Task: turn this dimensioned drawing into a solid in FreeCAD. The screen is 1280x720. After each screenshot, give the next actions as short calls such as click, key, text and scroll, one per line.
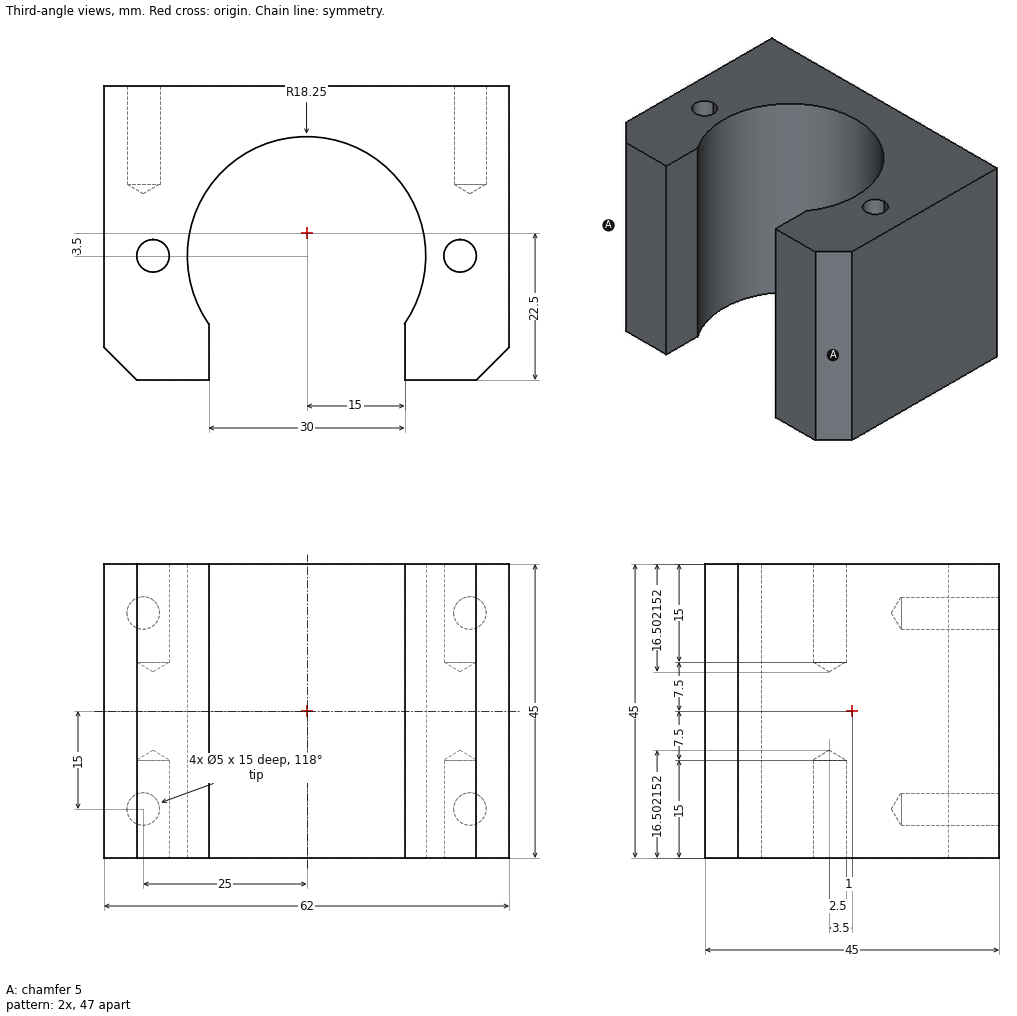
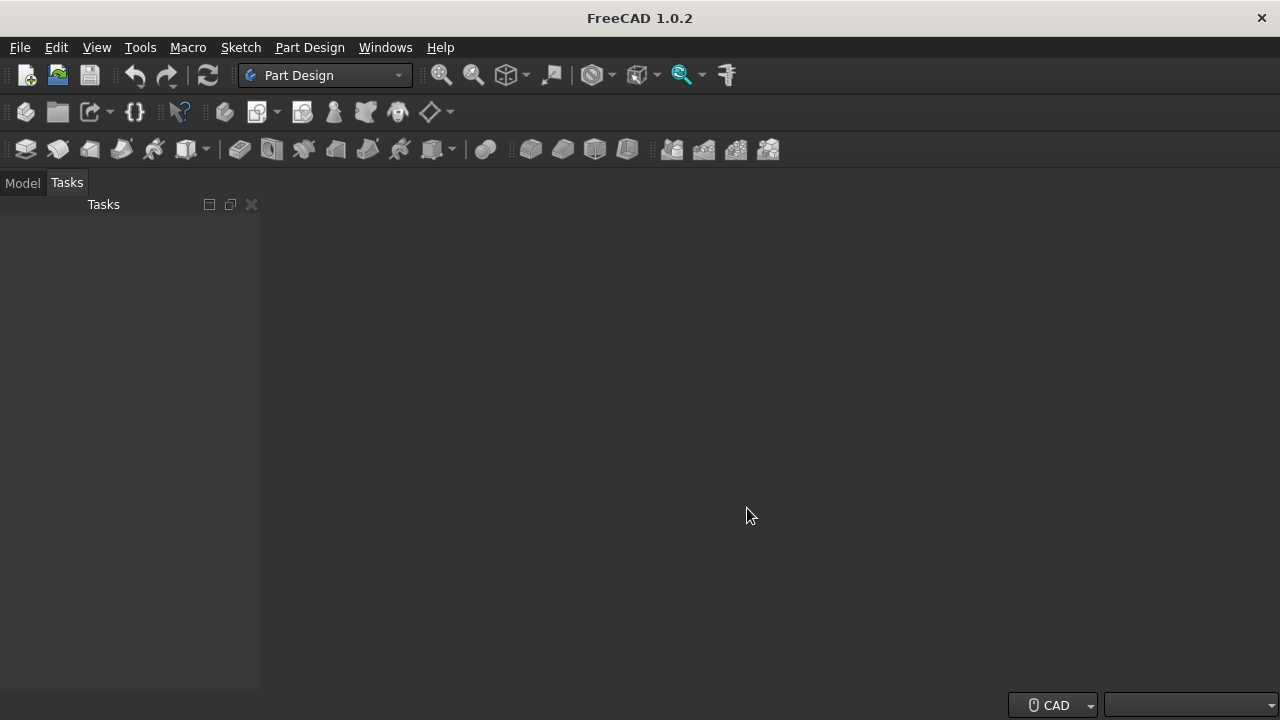
click(26, 76)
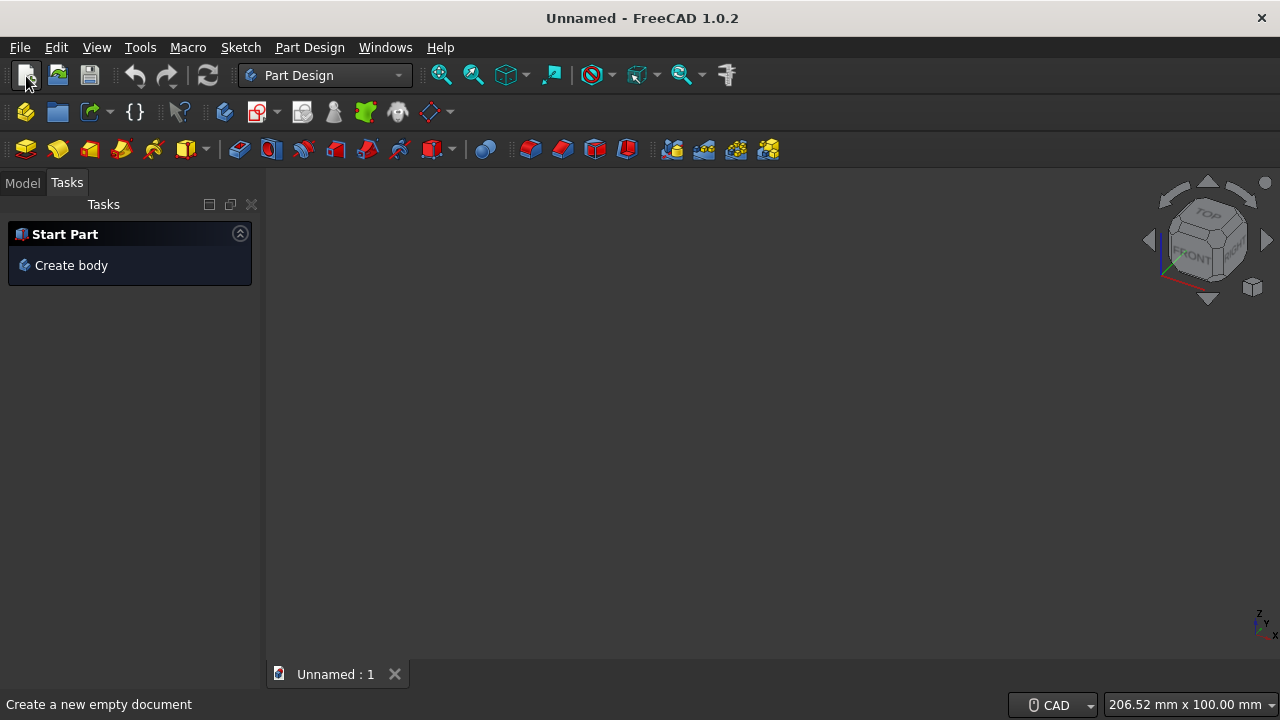
click(258, 112)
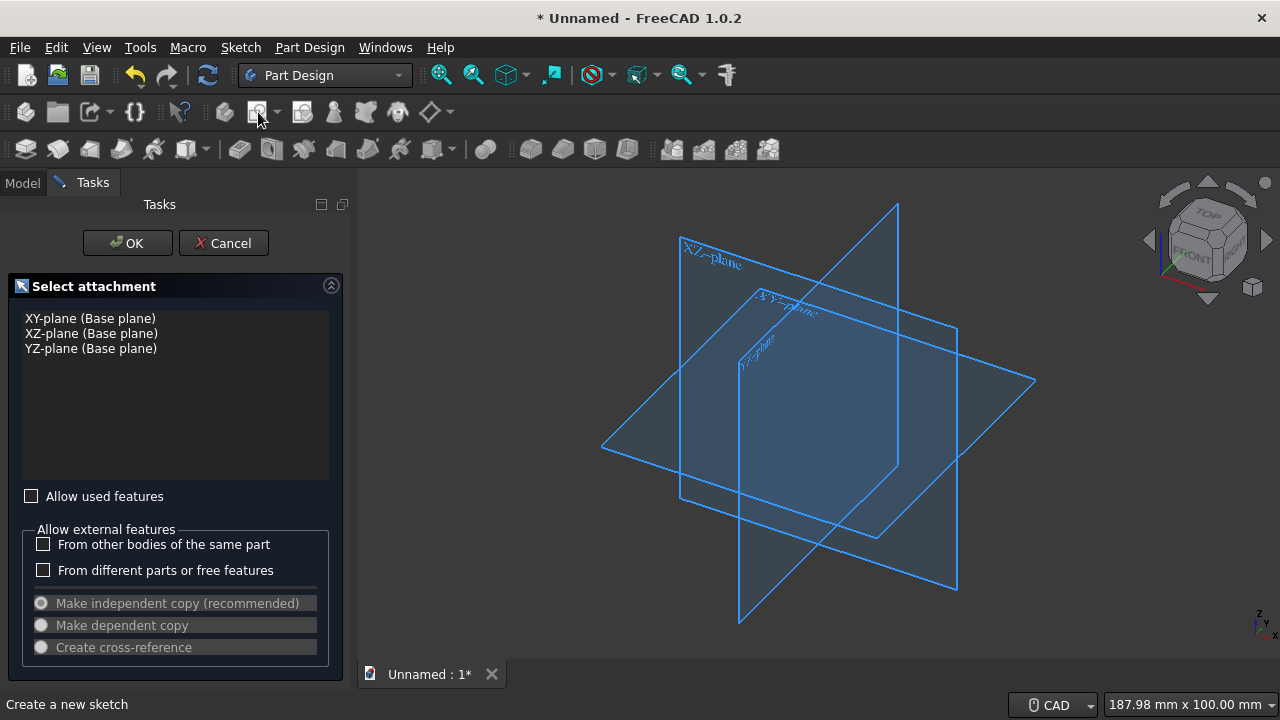
click(82, 334)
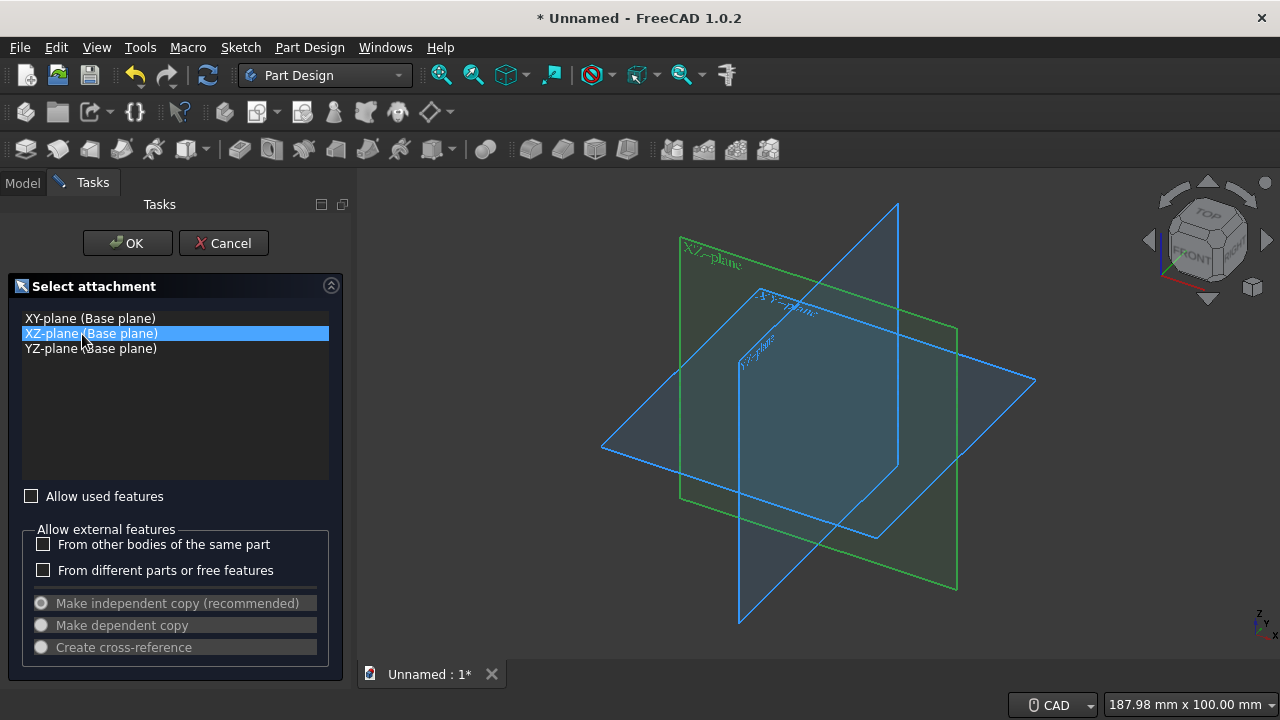
click(128, 243)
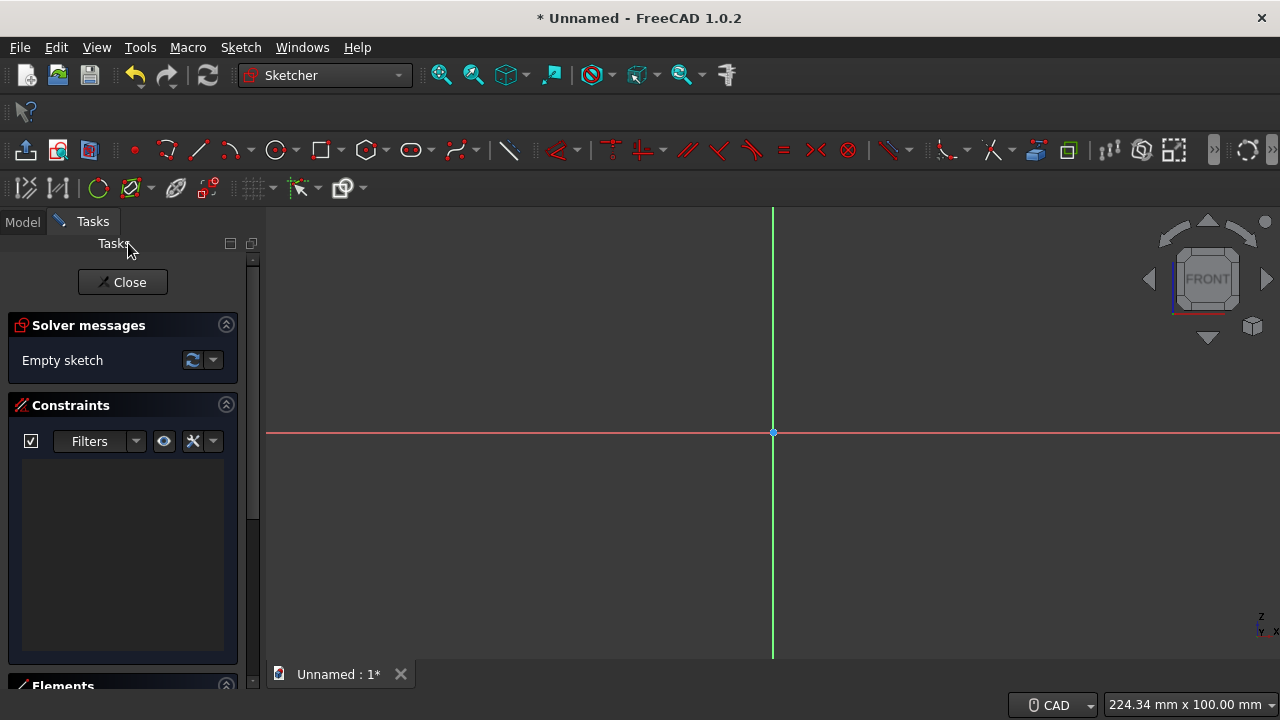
scroll(912, 433, up, 2)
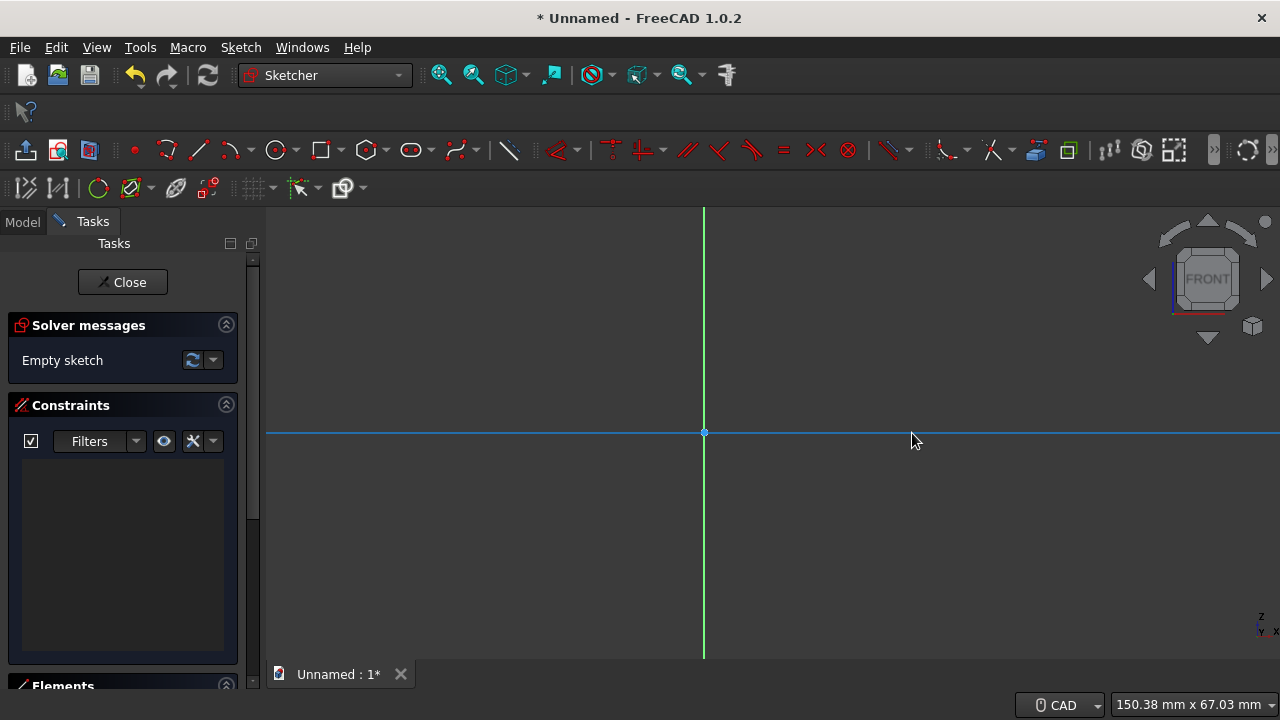
key(g)
key(v)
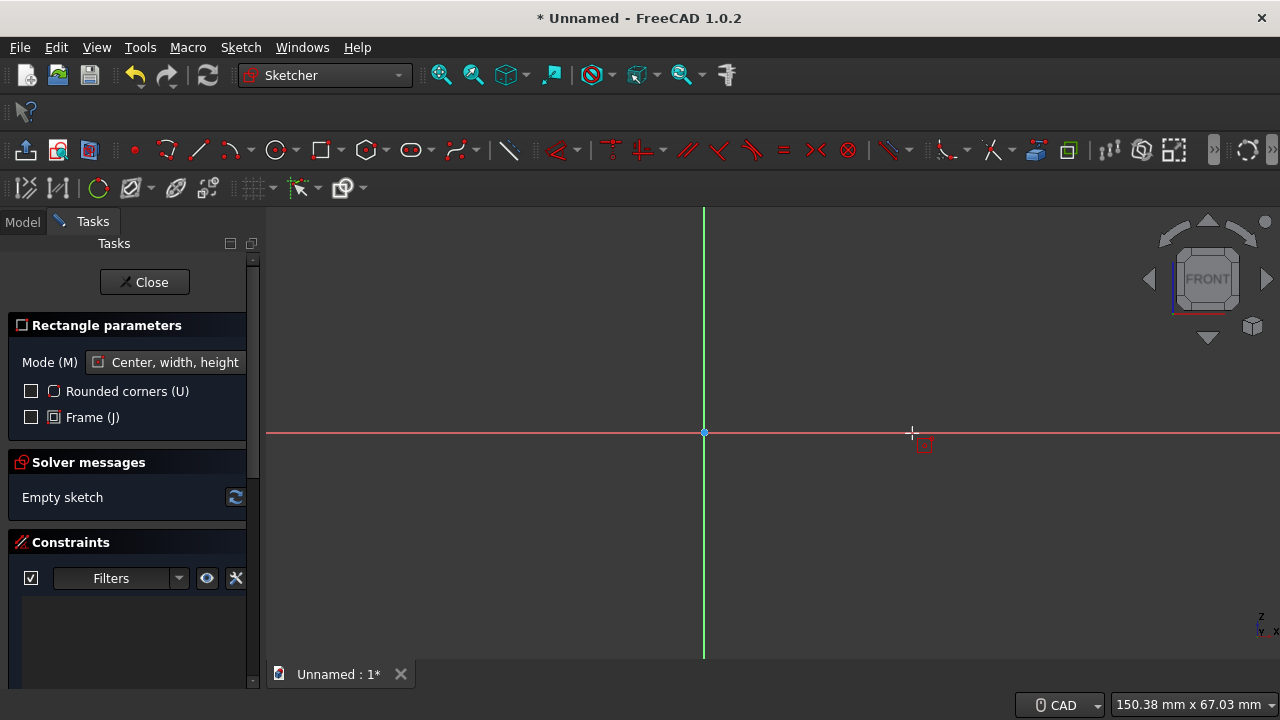
click(704, 433)
click(913, 281)
key(Escape)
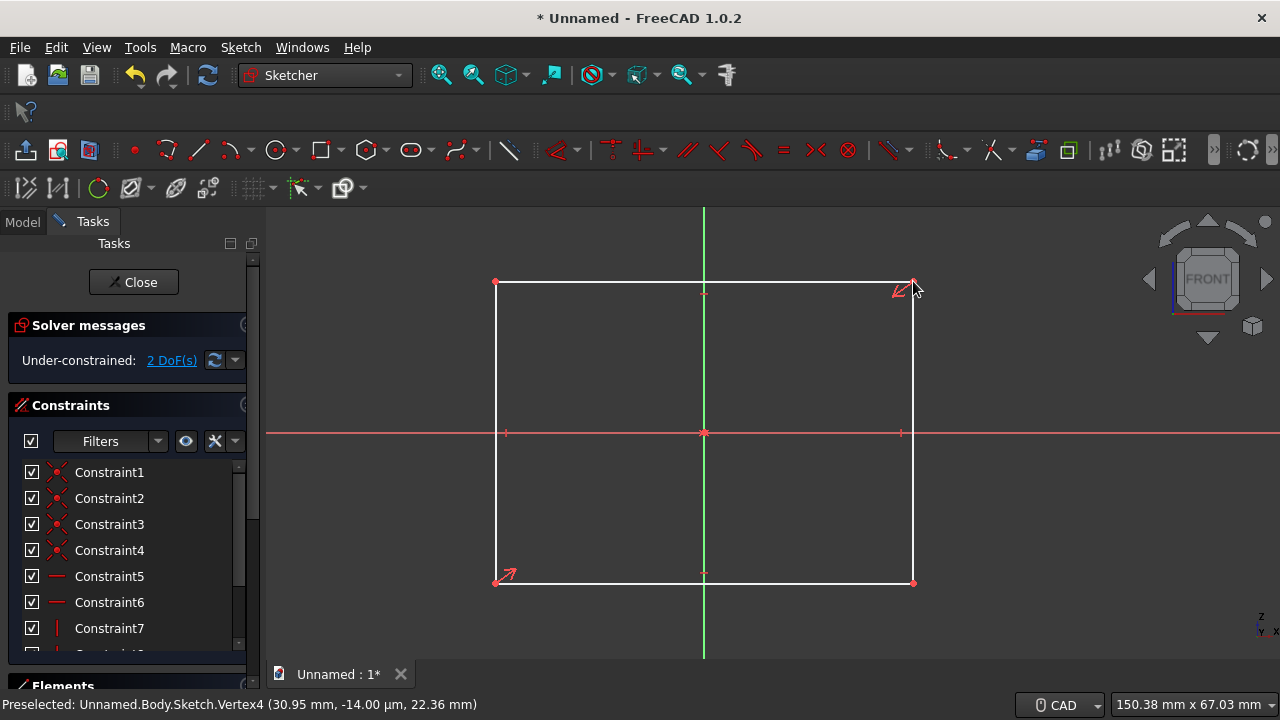
click(556, 150)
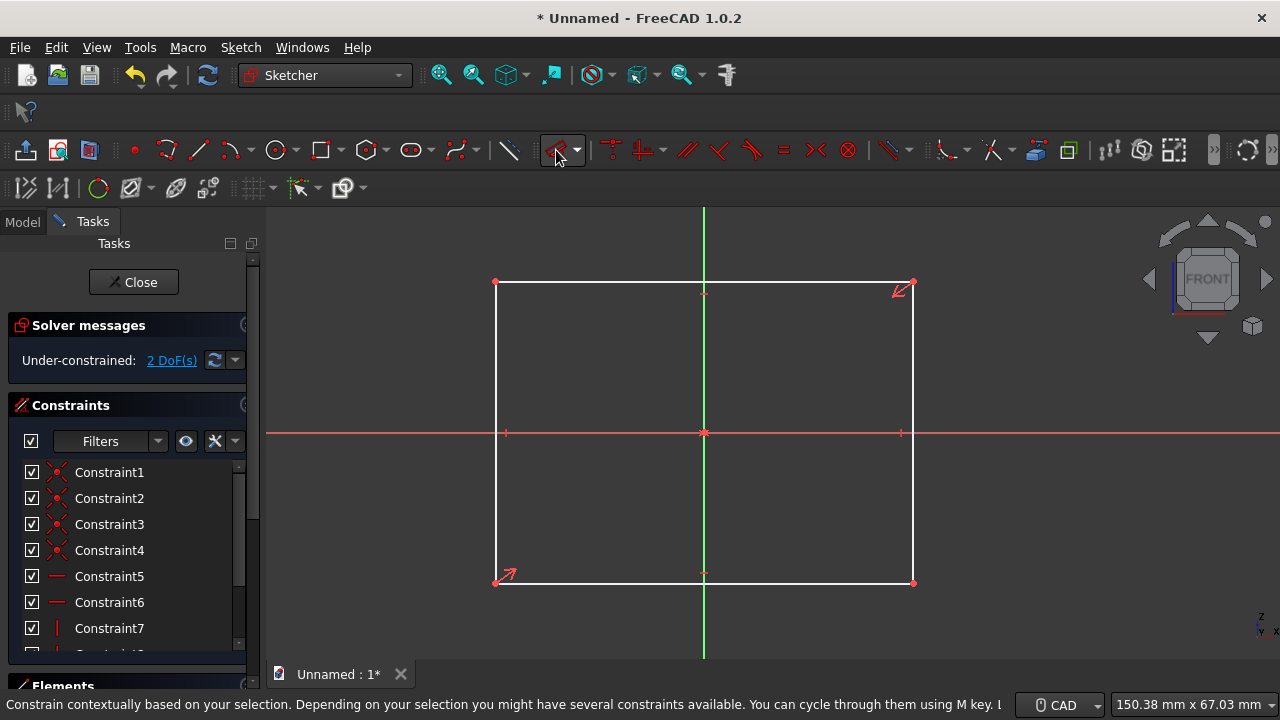
click(621, 584)
click(608, 618)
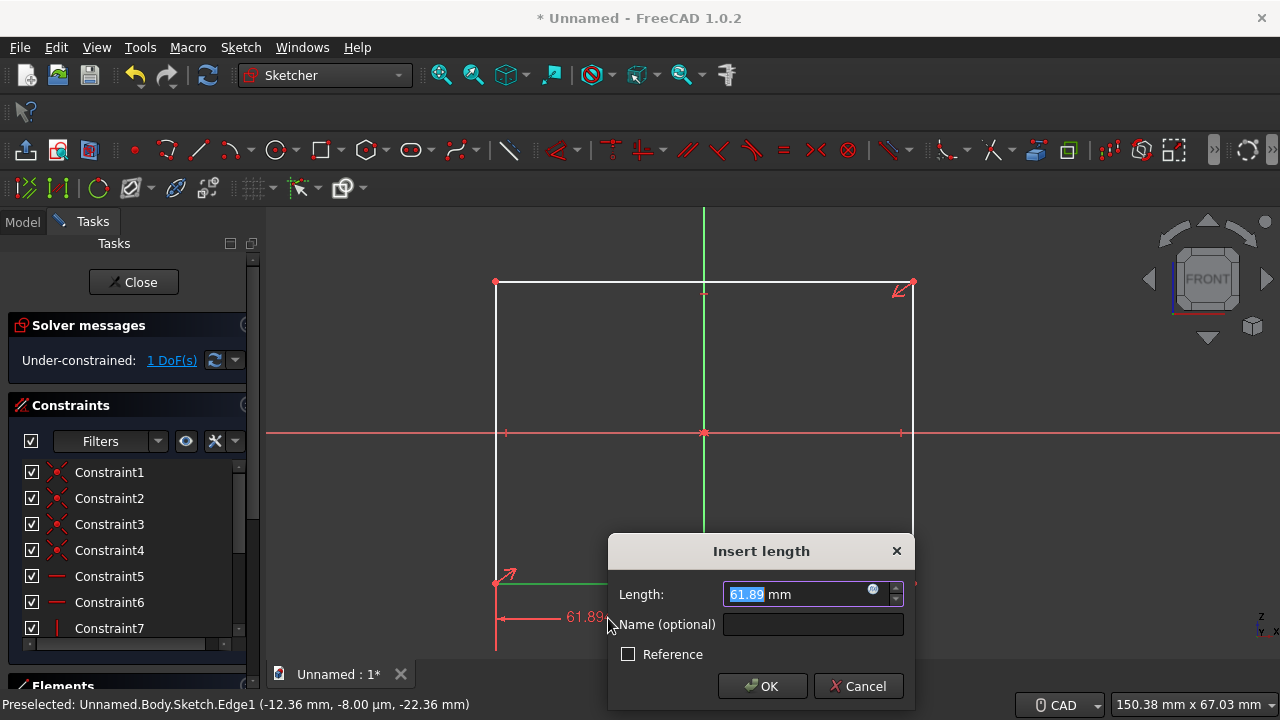
text(62)
key(Return)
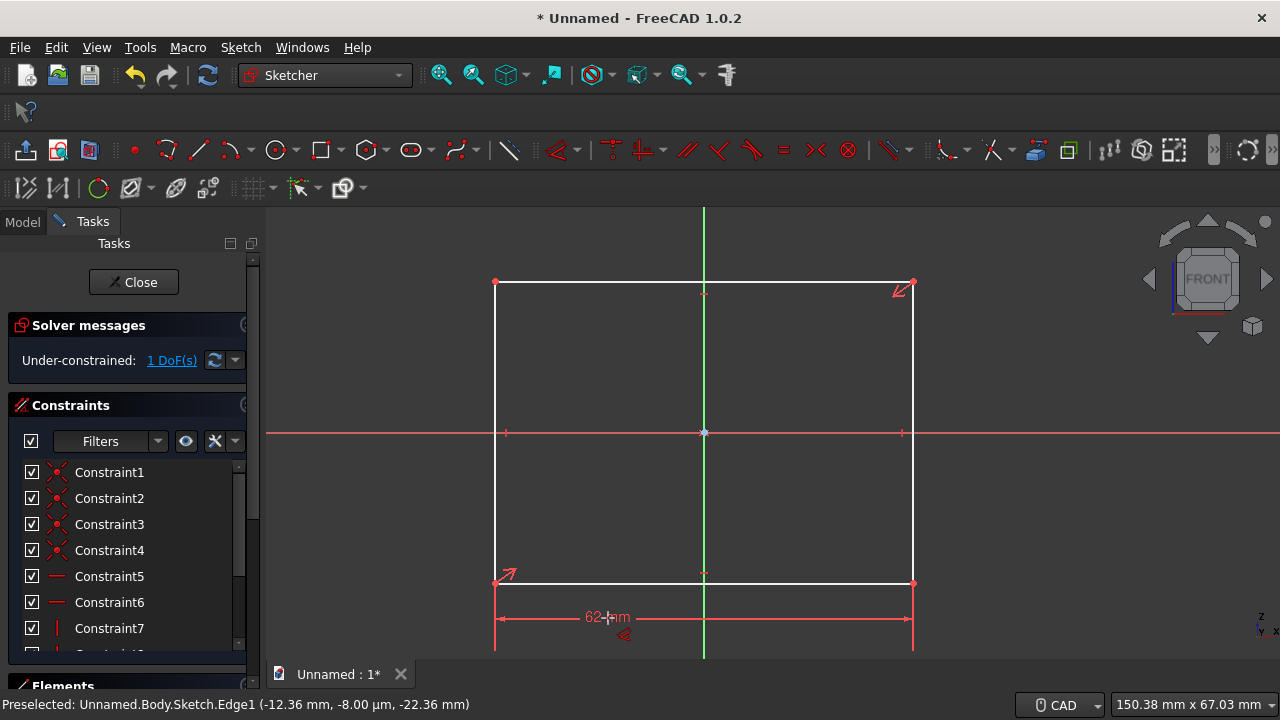
click(913, 493)
click(947, 363)